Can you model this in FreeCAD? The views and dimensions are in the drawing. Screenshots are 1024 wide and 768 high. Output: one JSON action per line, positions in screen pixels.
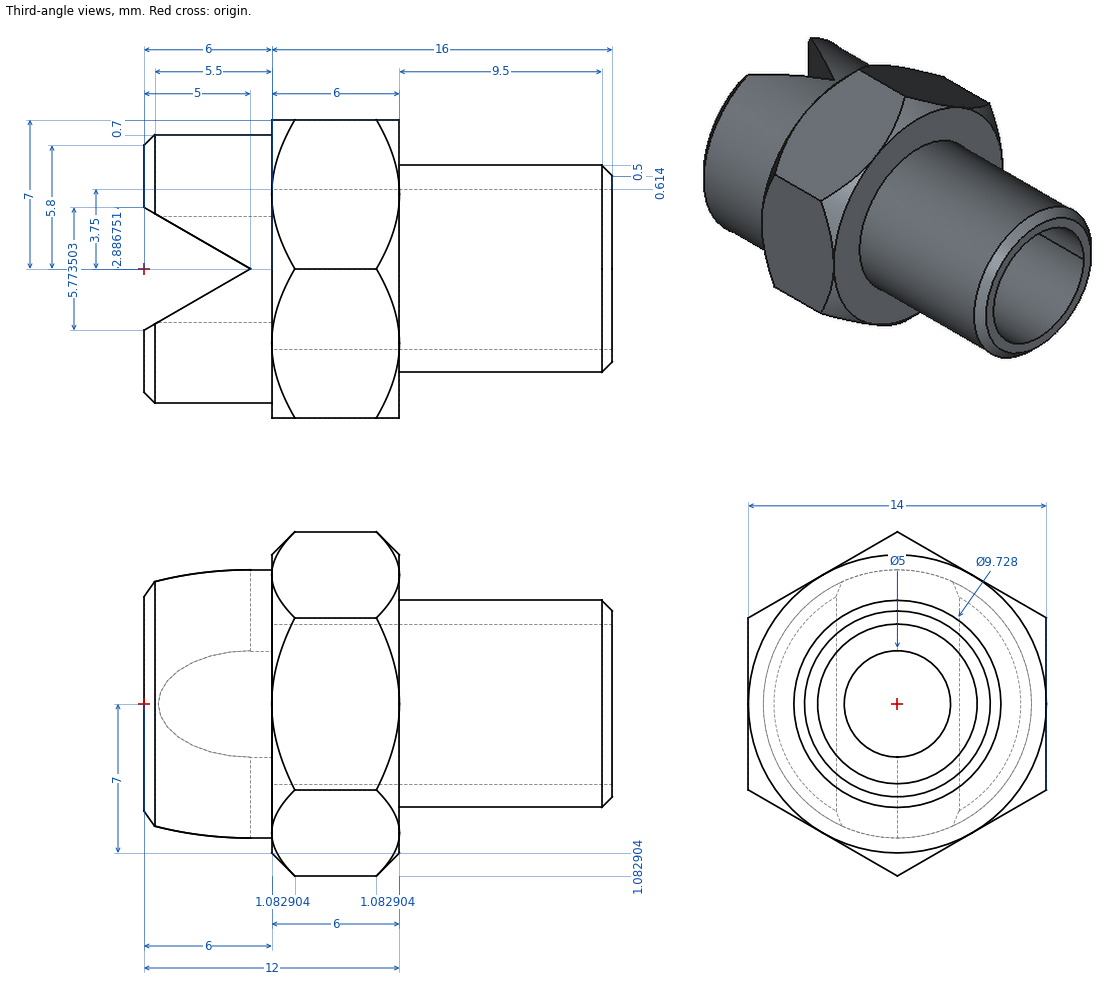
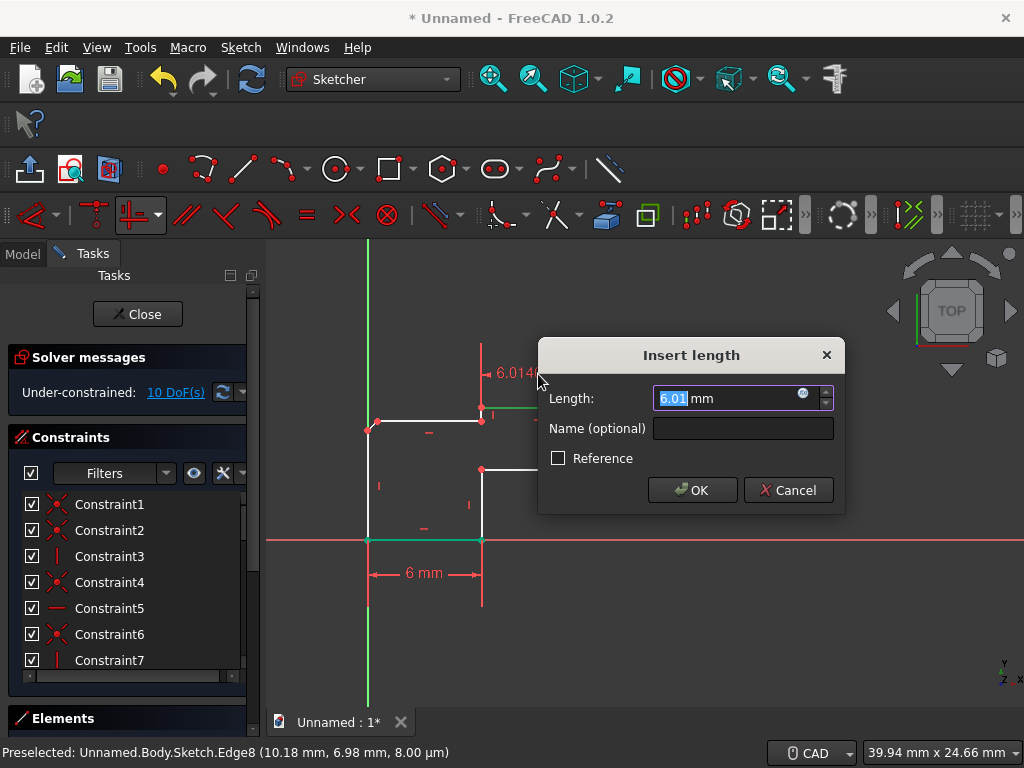
{"action": "type", "text": "6"}
{"action": "key", "text": "Return"}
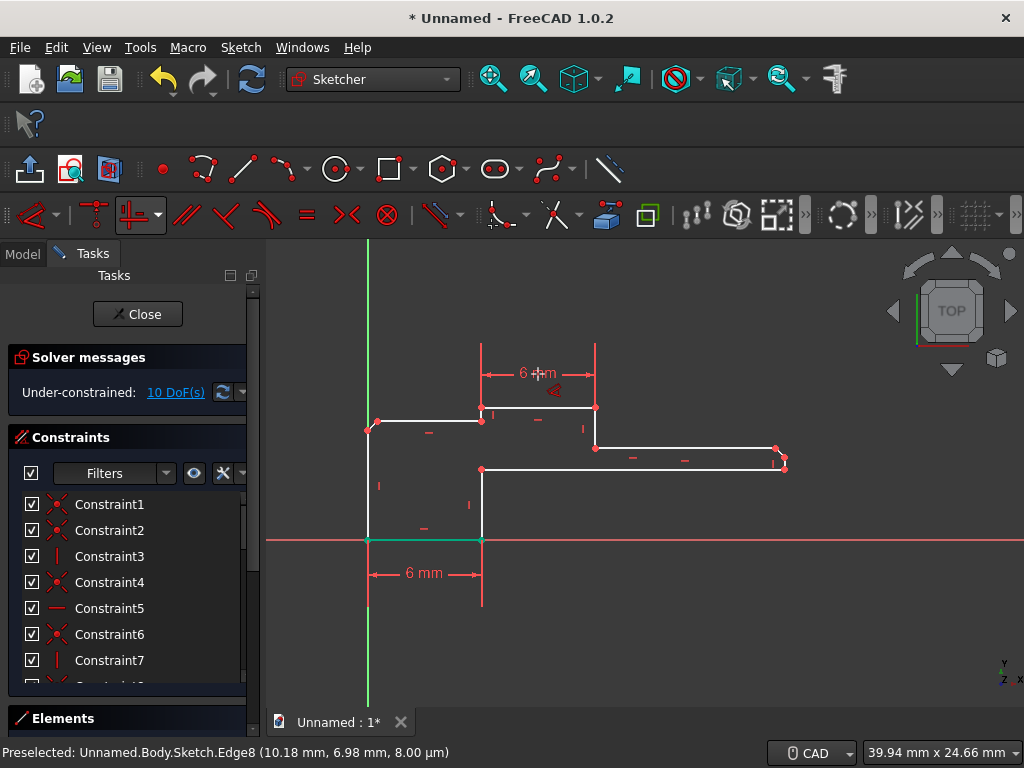
{"action": "left_click", "coordinate": [573, 470]}
{"action": "left_click", "coordinate": [563, 436]}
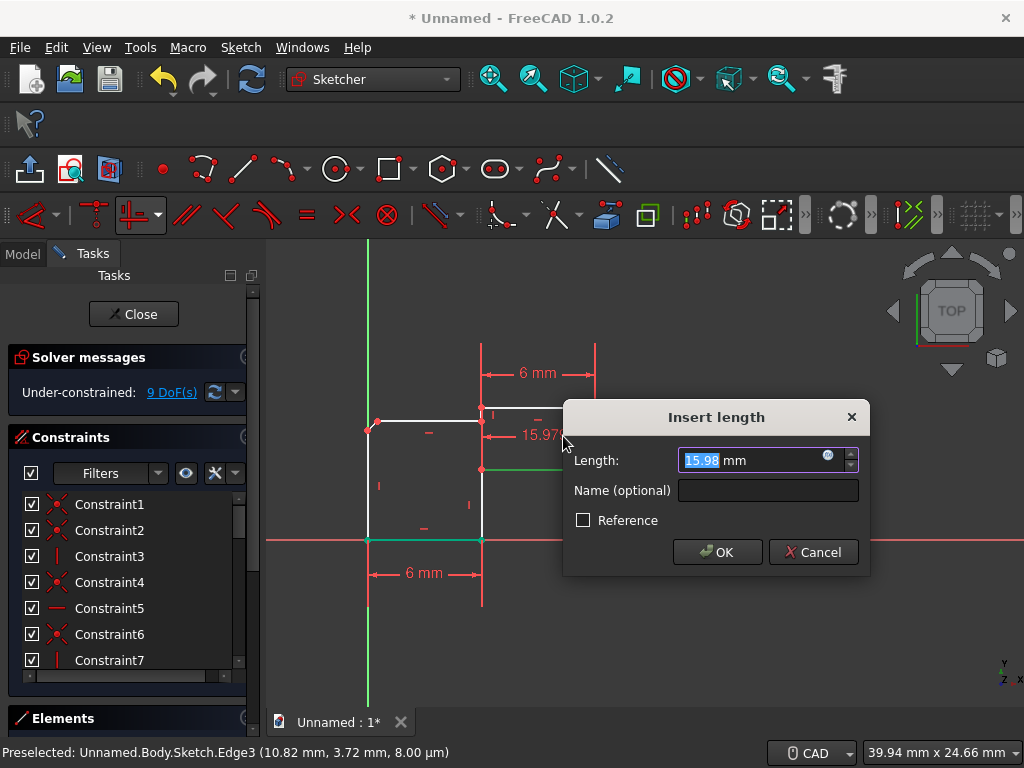
{"action": "type", "text": "16"}
{"action": "key", "text": "Return"}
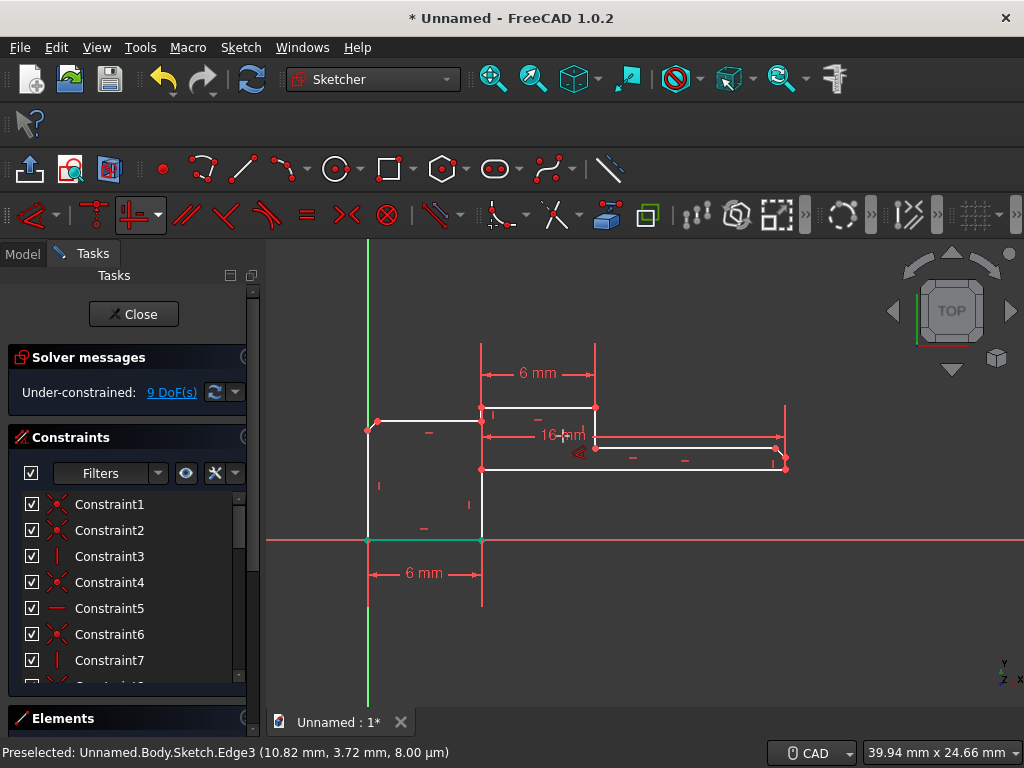
{"action": "left_click", "coordinate": [595, 408]}
{"action": "left_click", "coordinate": [334, 474]}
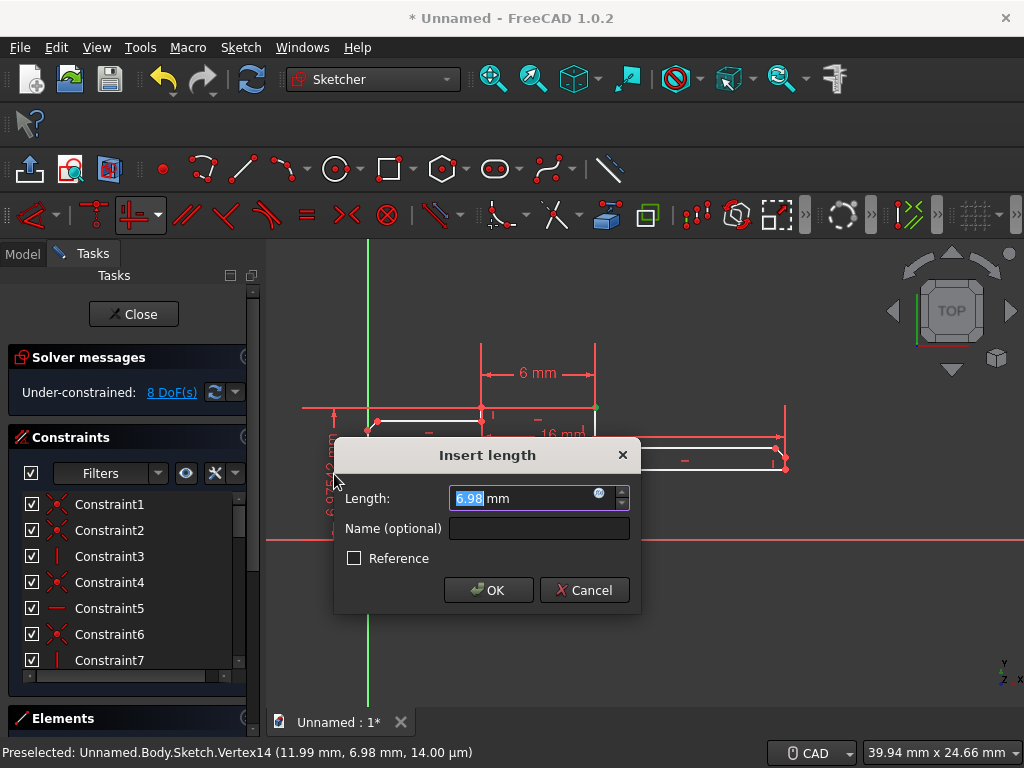
{"action": "type", "text": "7"}
{"action": "key", "text": "Return"}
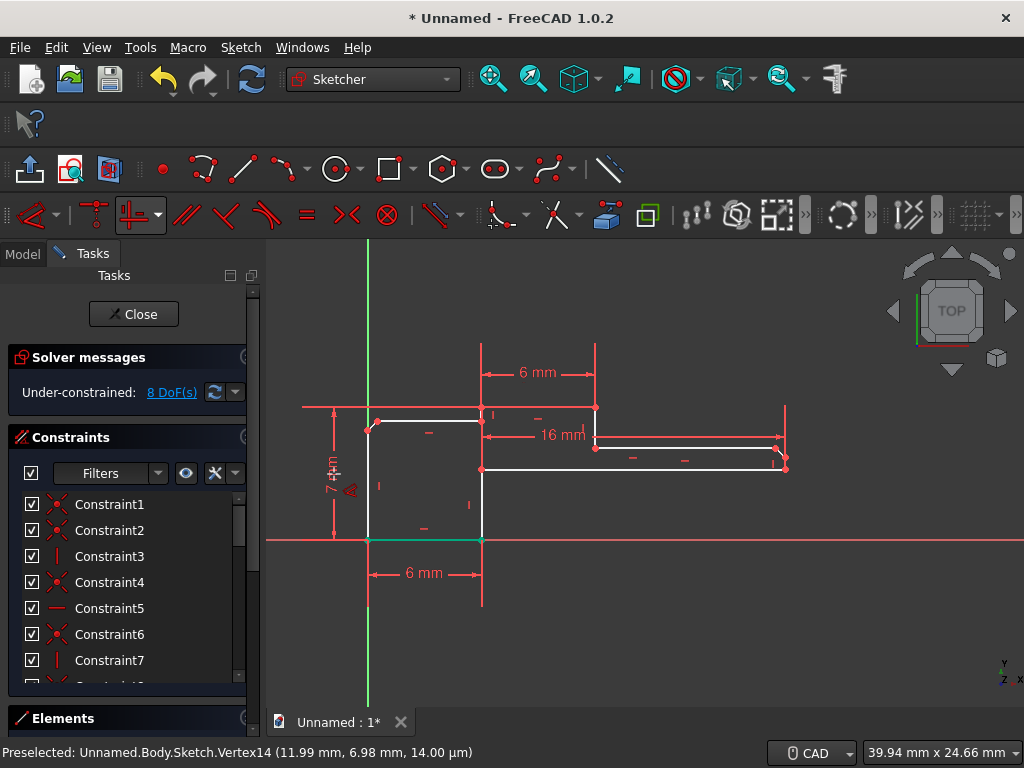
{"action": "left_click", "coordinate": [481, 407]}
{"action": "left_click", "coordinate": [425, 373]}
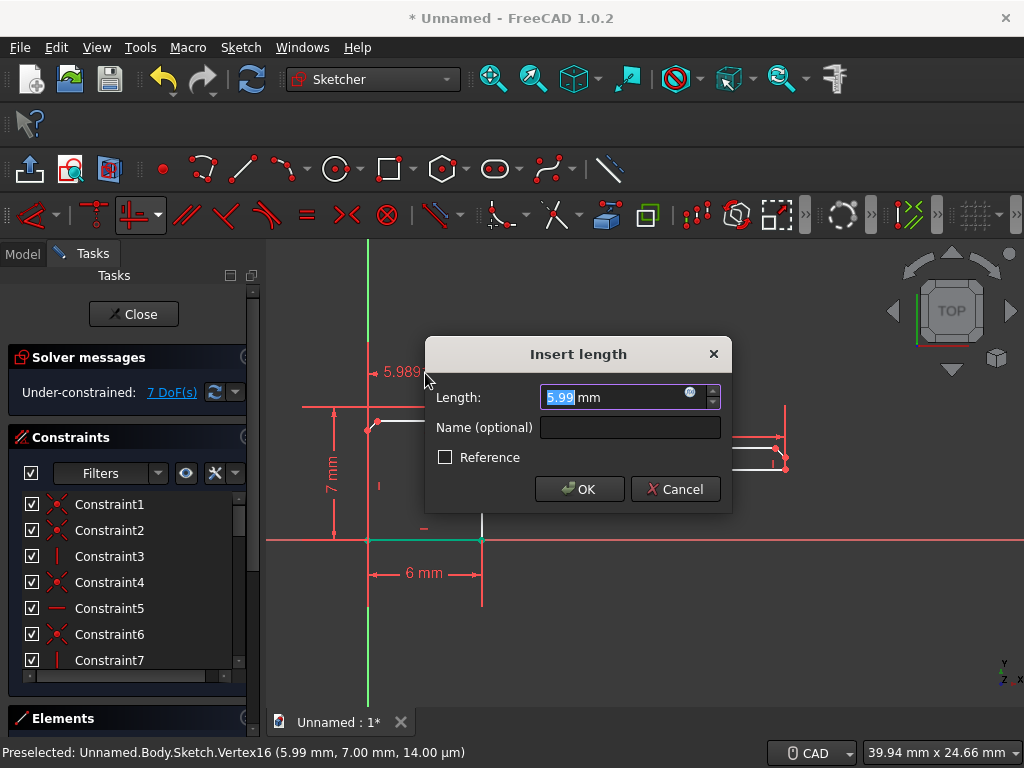
{"action": "type", "text": "6"}
{"action": "key", "text": "Return"}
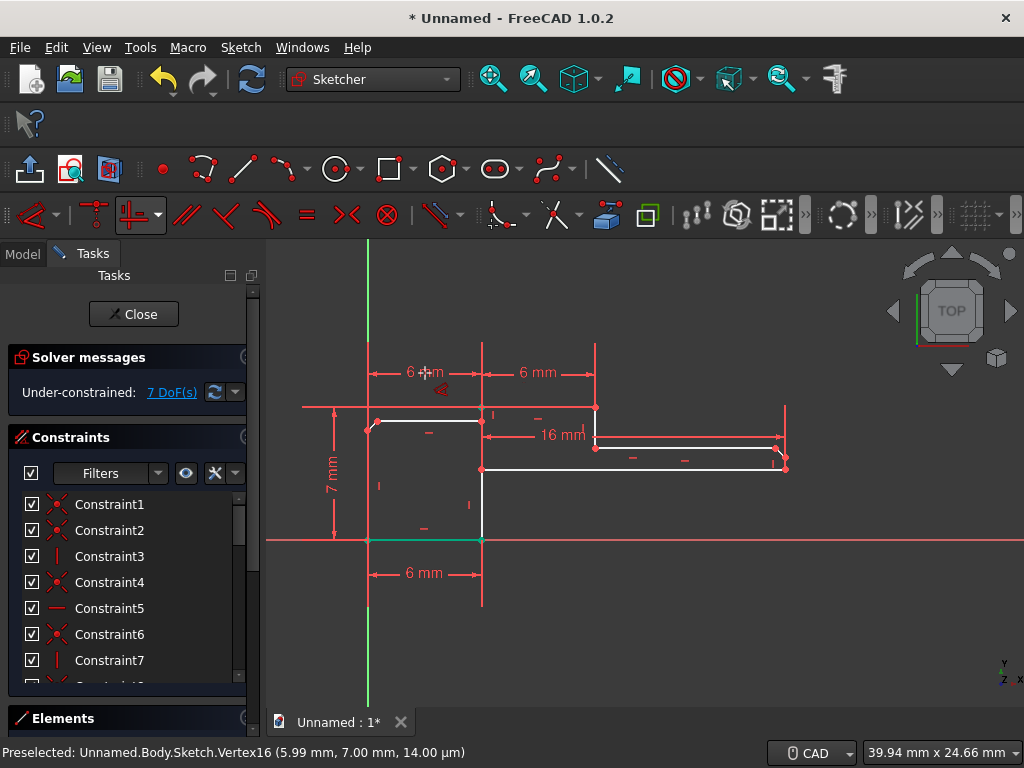
{"action": "left_click", "coordinate": [722, 448]}
{"action": "left_click", "coordinate": [686, 414]}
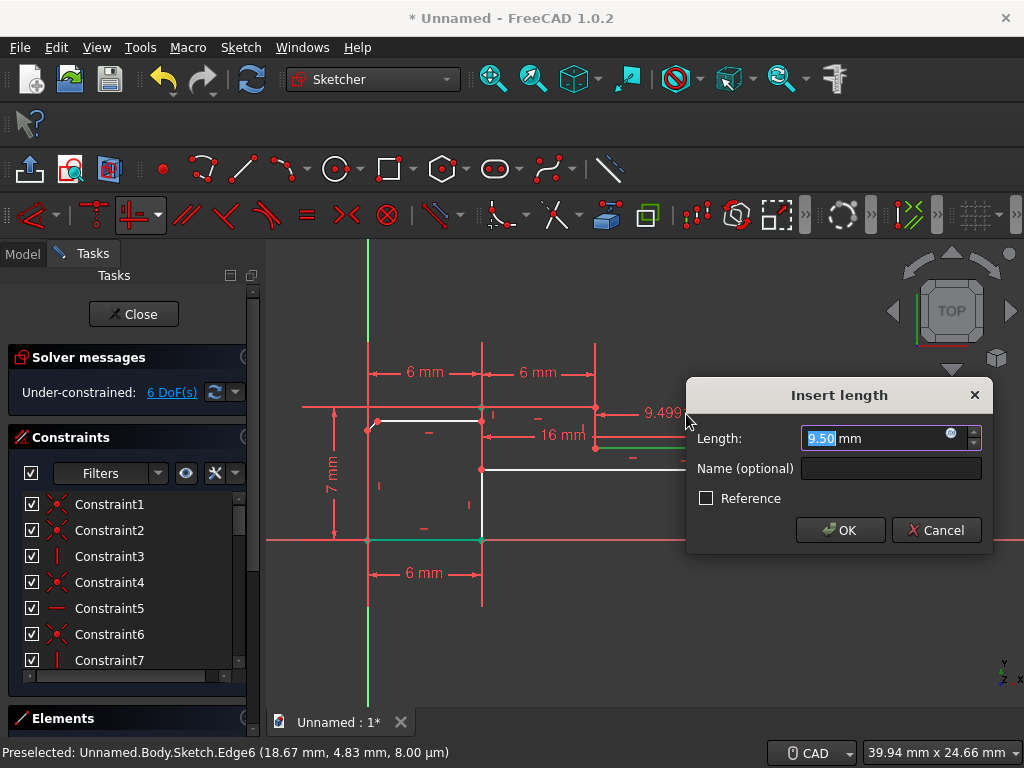
{"action": "type", "text": "9.5"}
{"action": "key", "text": "Return"}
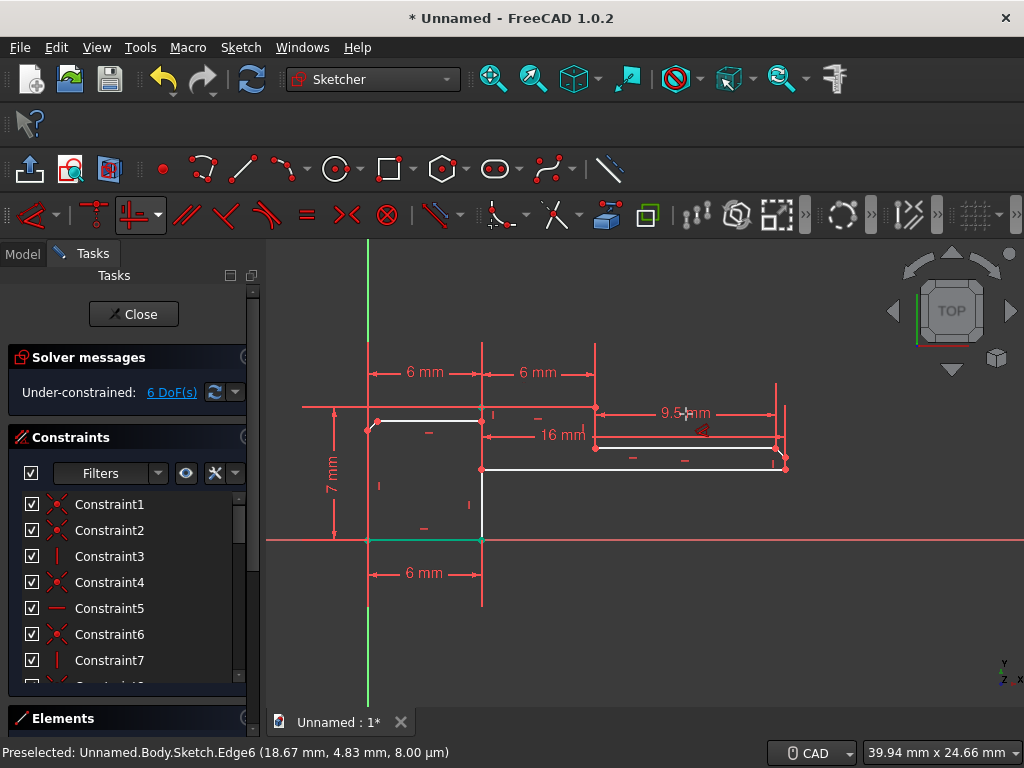
{"action": "scroll", "coordinate": [482, 414], "scroll_direction": "up", "scroll_amount": 6}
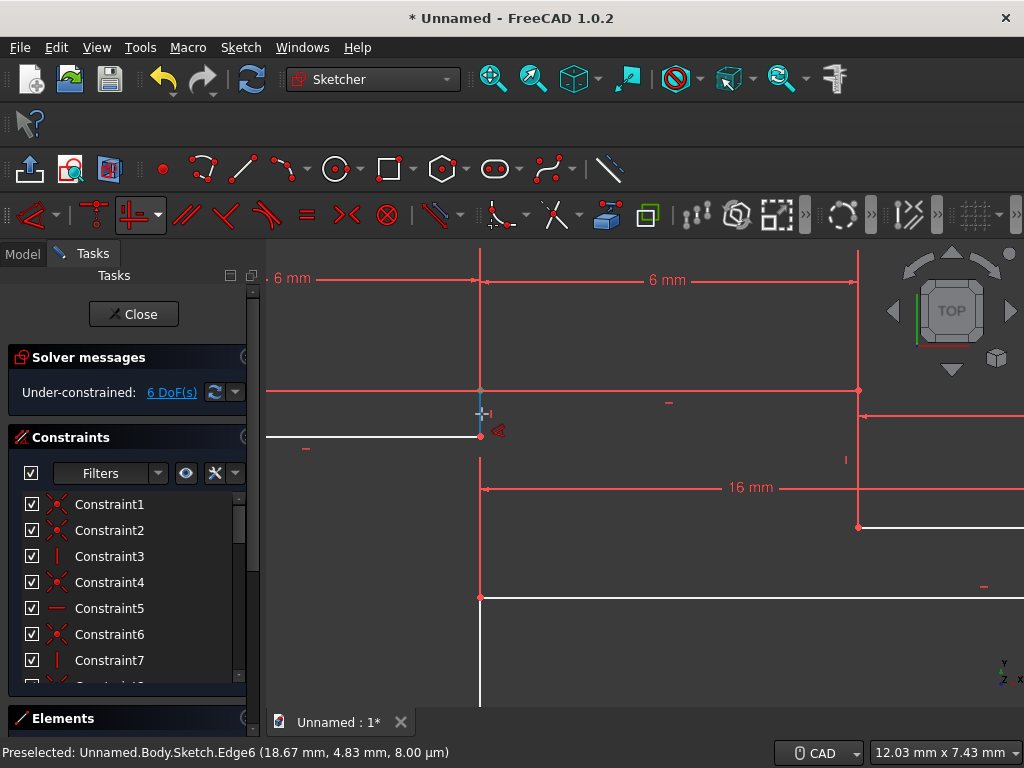
{"action": "left_click", "coordinate": [480, 414]}
{"action": "left_click", "coordinate": [446, 414]}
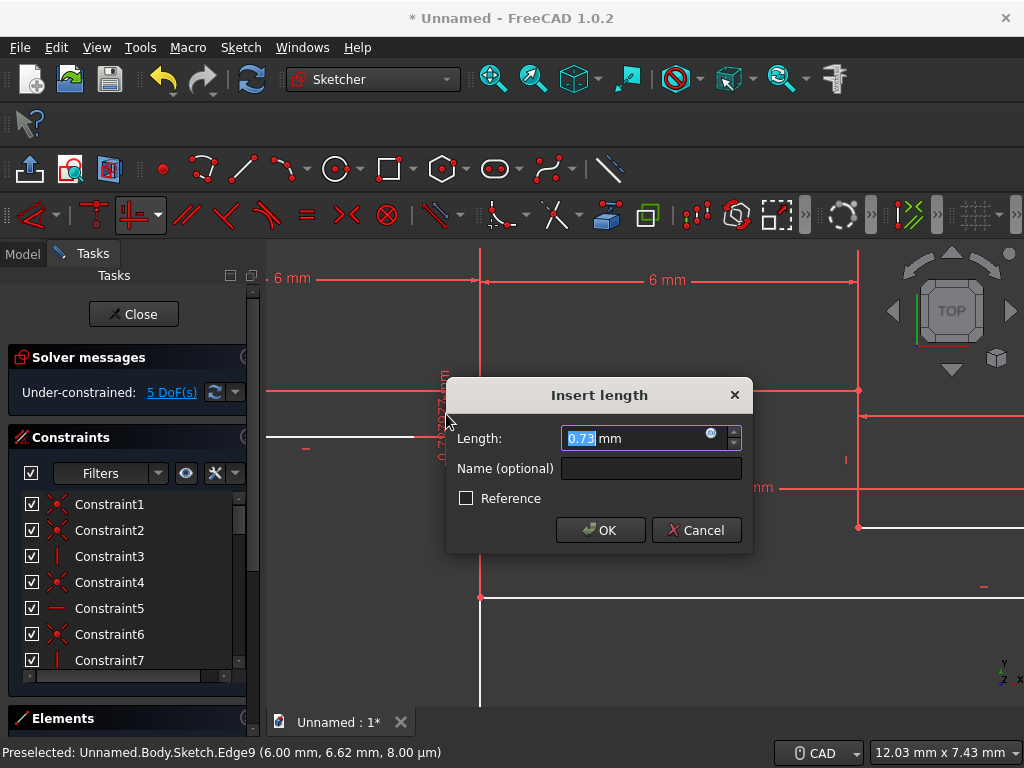
{"action": "type", "text": "0.7"}
{"action": "key", "text": "Return"}